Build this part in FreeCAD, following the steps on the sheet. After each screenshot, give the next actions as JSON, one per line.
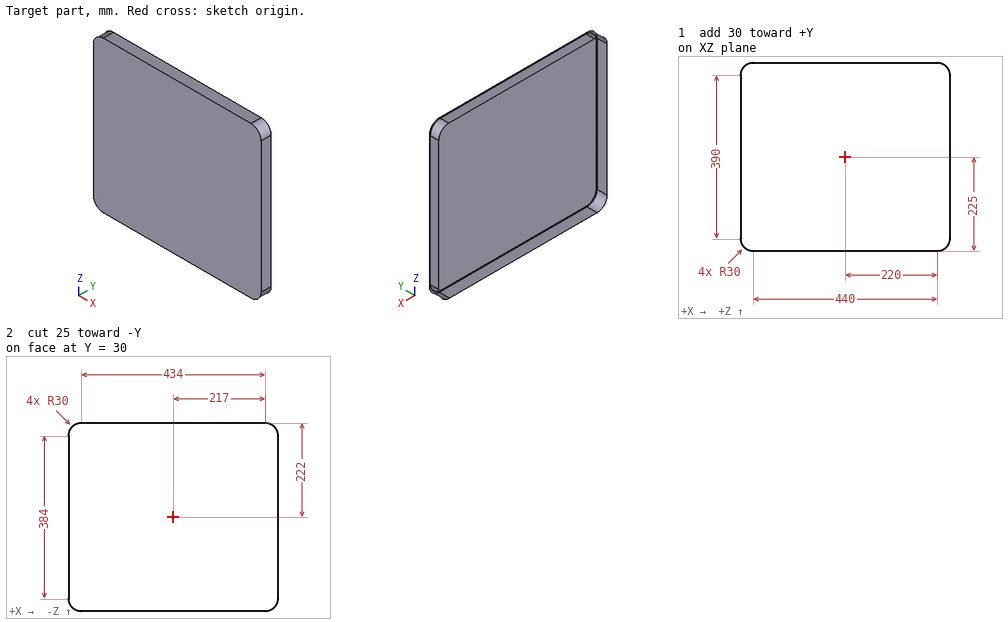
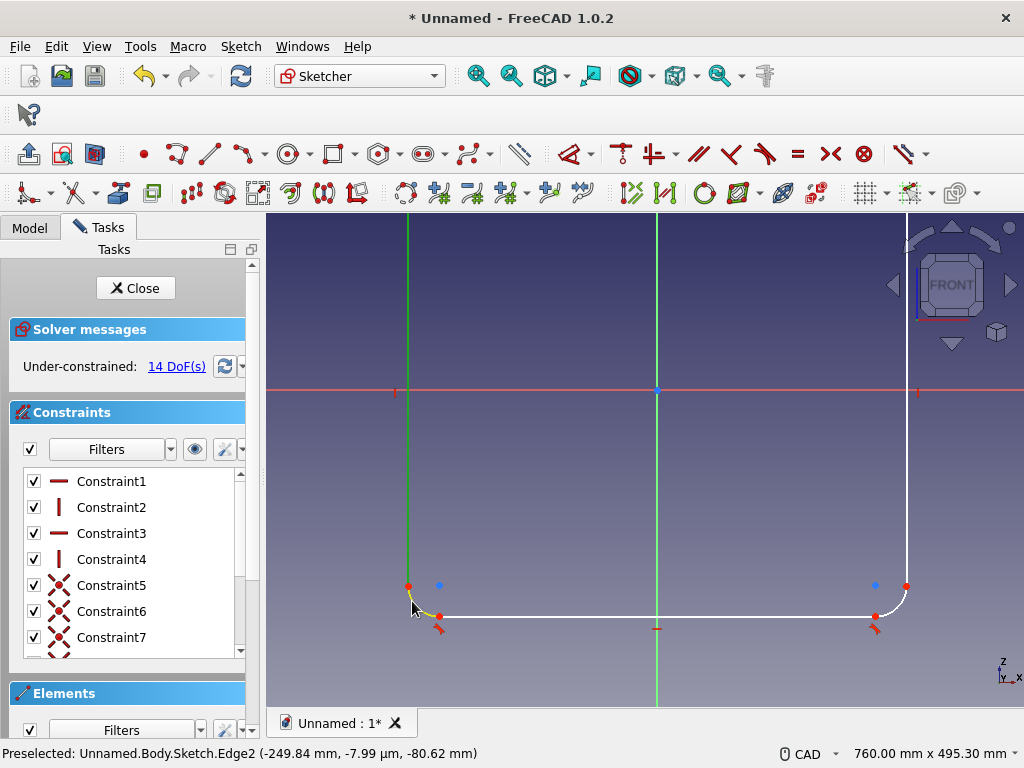
{"action": "left_click", "coordinate": [412, 600]}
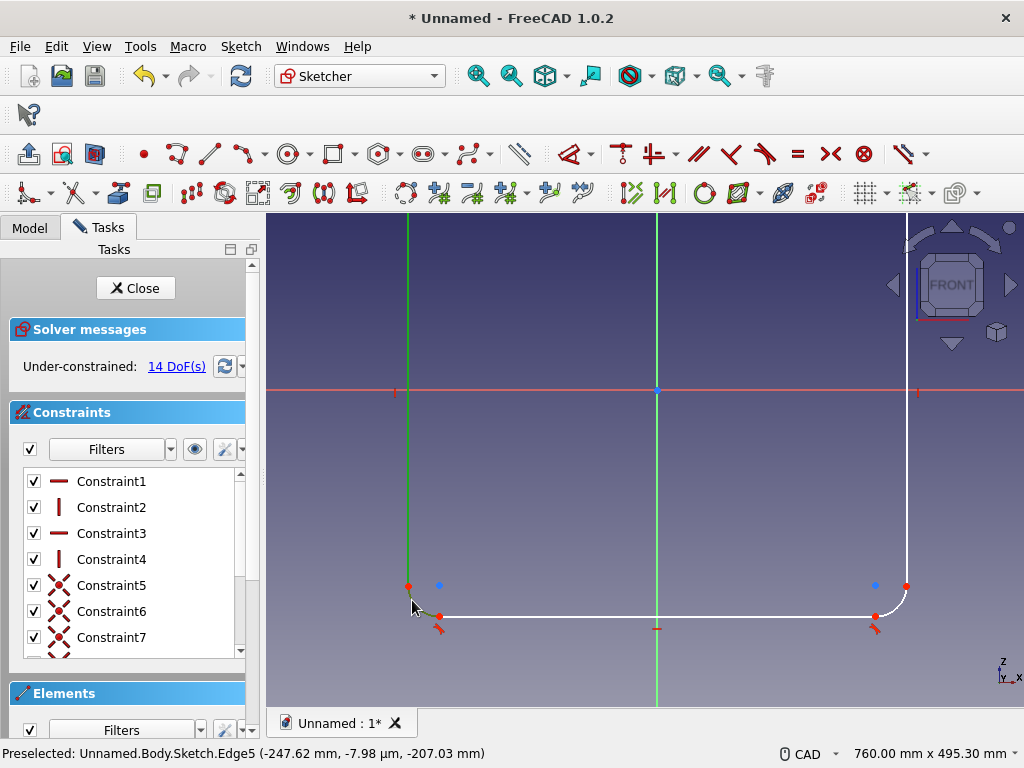
{"action": "left_click", "coordinate": [765, 154]}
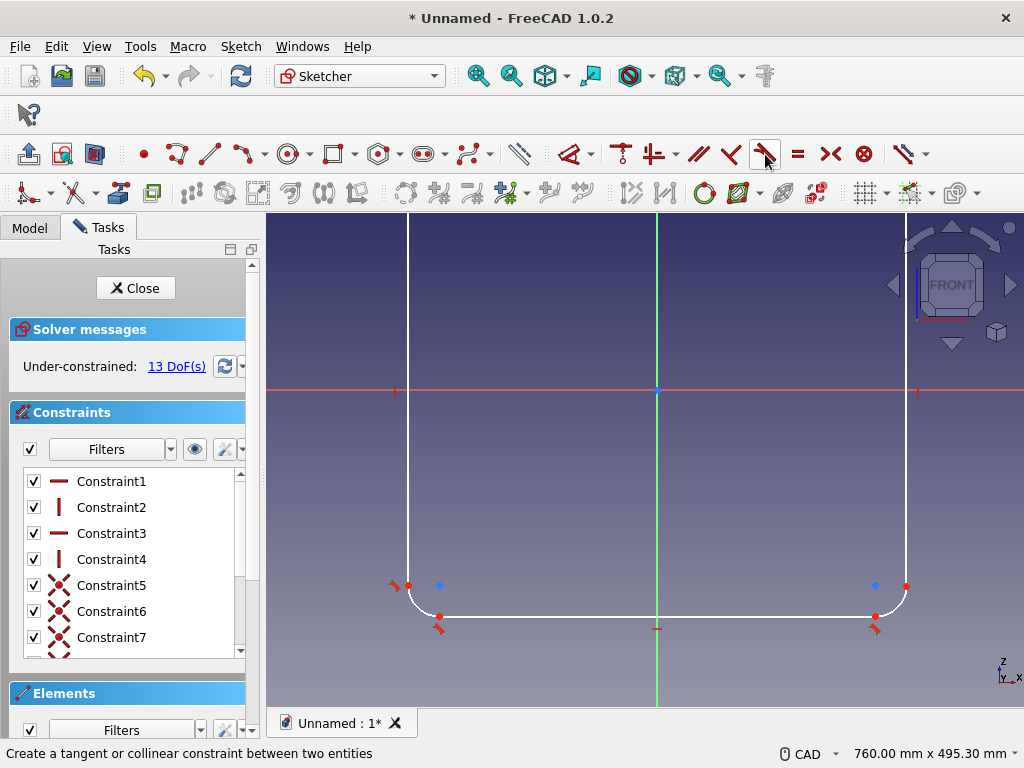
{"action": "left_click", "coordinate": [408, 469]}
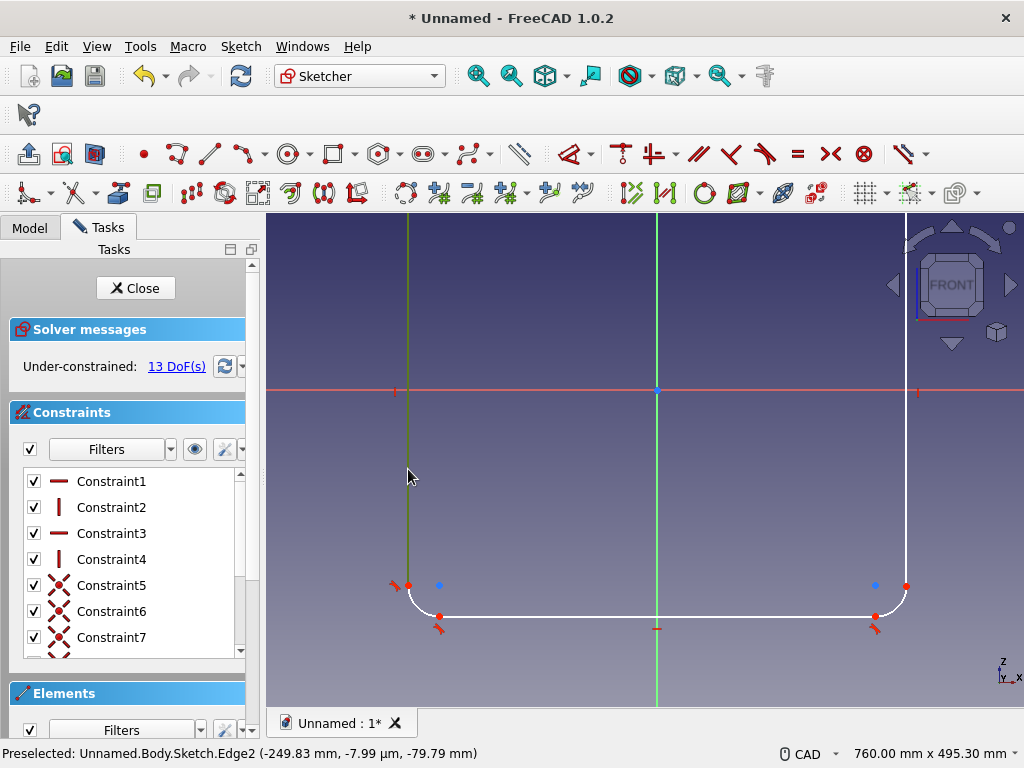
{"action": "scroll", "coordinate": [412, 601], "scroll_direction": "down", "scroll_amount": 2}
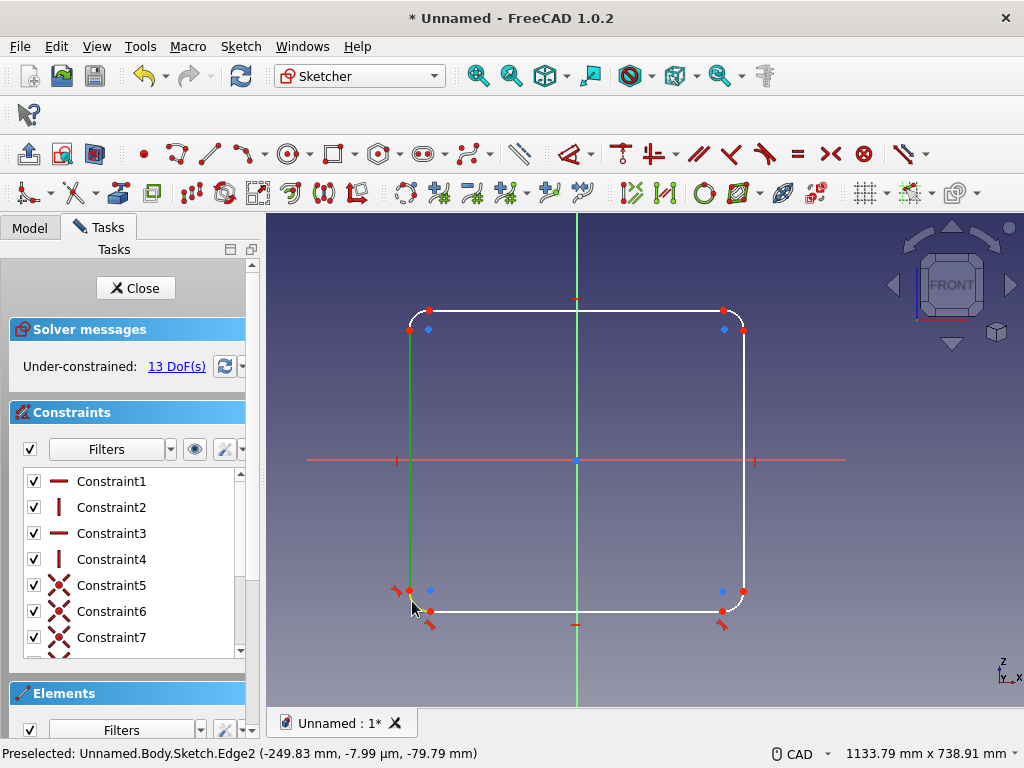
{"action": "scroll", "coordinate": [420, 312], "scroll_direction": "up", "scroll_amount": 2}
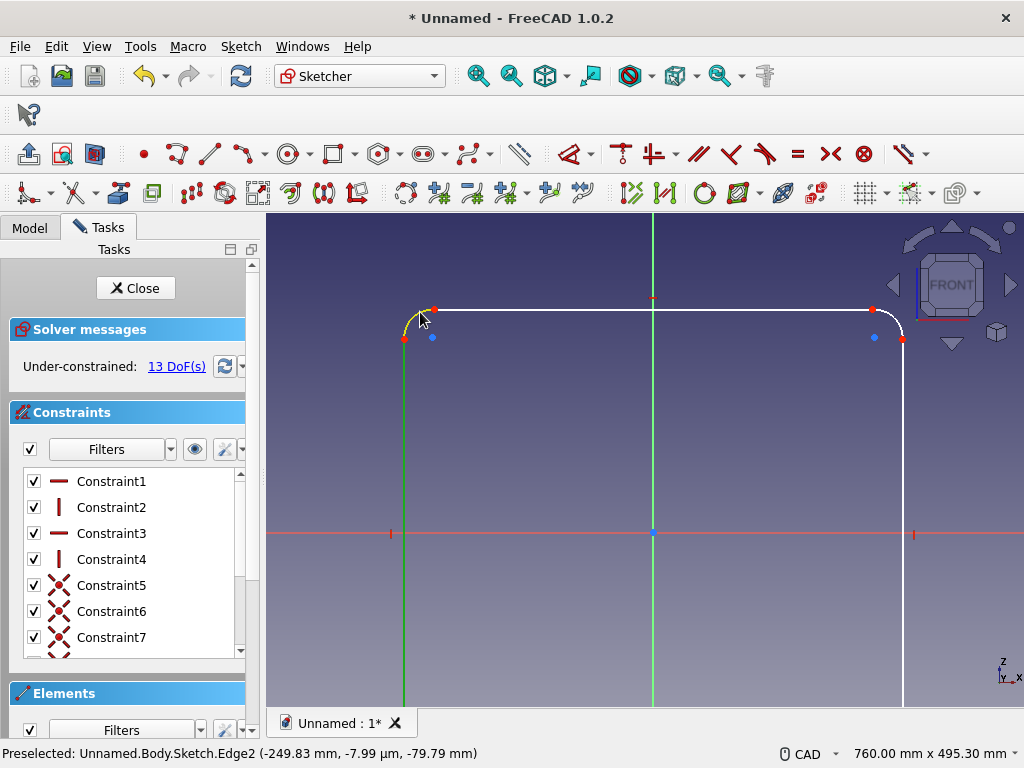
{"action": "left_click", "coordinate": [420, 313]}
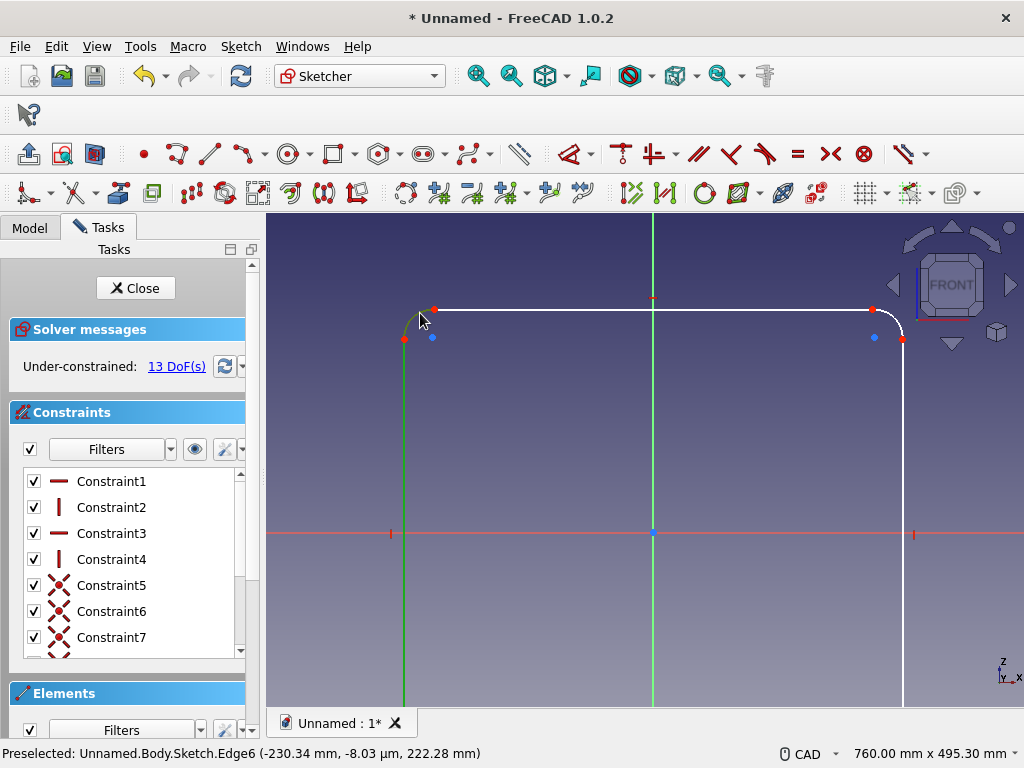
{"action": "left_click", "coordinate": [765, 154]}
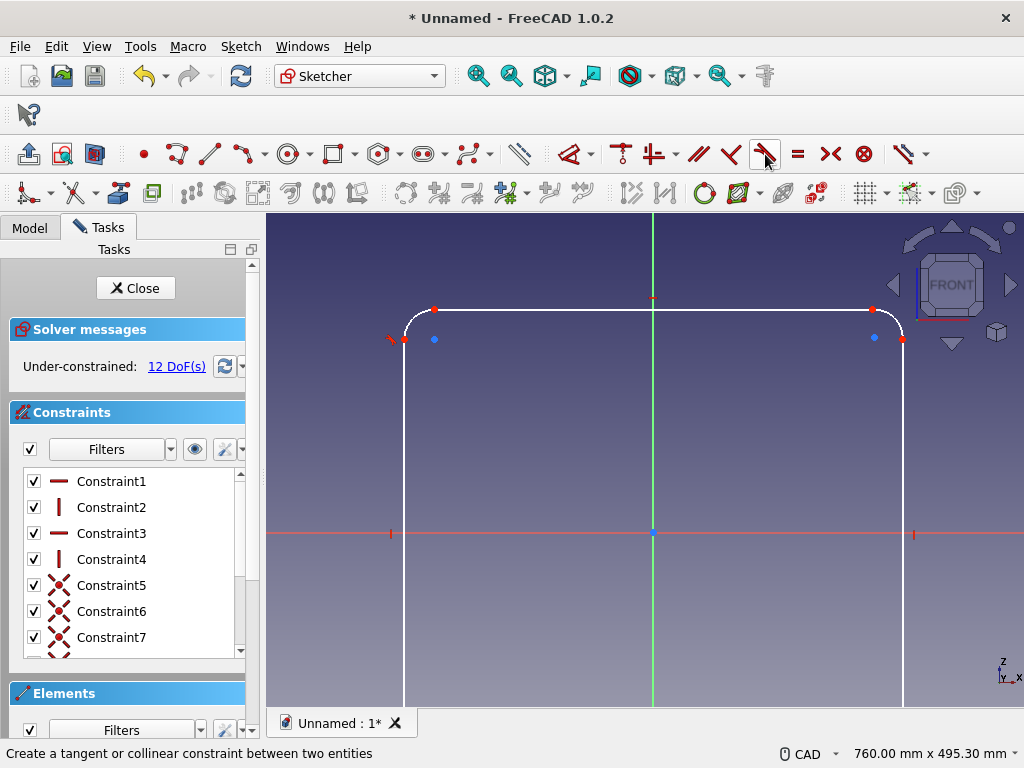
{"action": "left_click", "coordinate": [566, 310]}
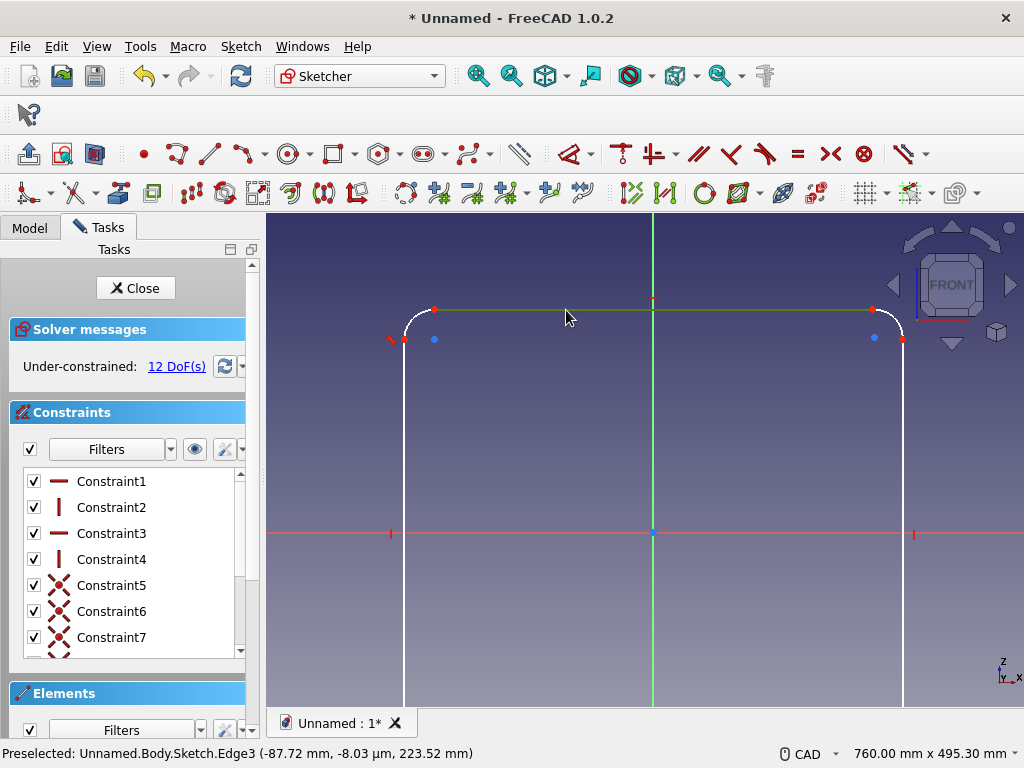
{"action": "left_click", "coordinate": [421, 313]}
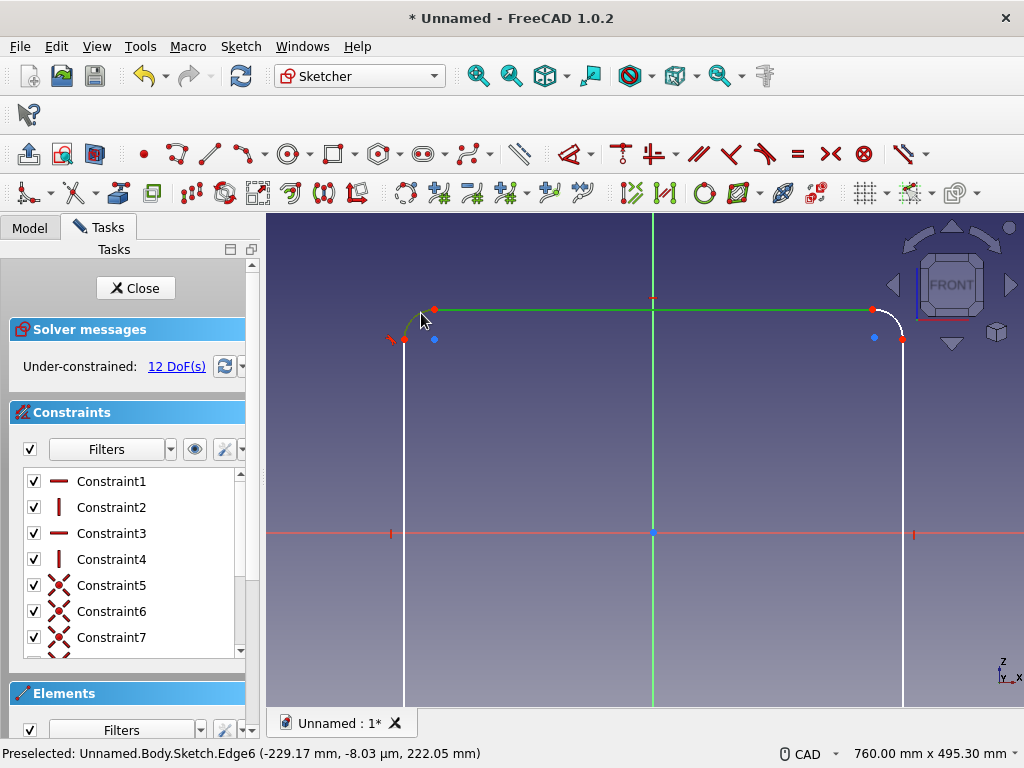
{"action": "left_click", "coordinate": [765, 154]}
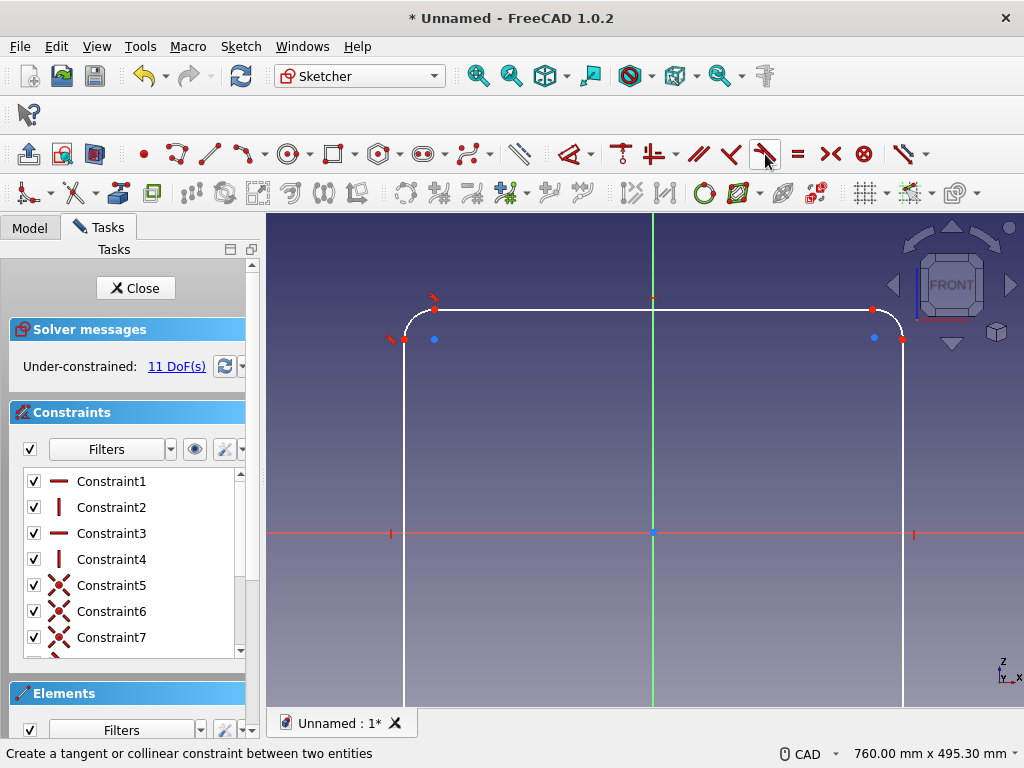
{"action": "left_click", "coordinate": [566, 310]}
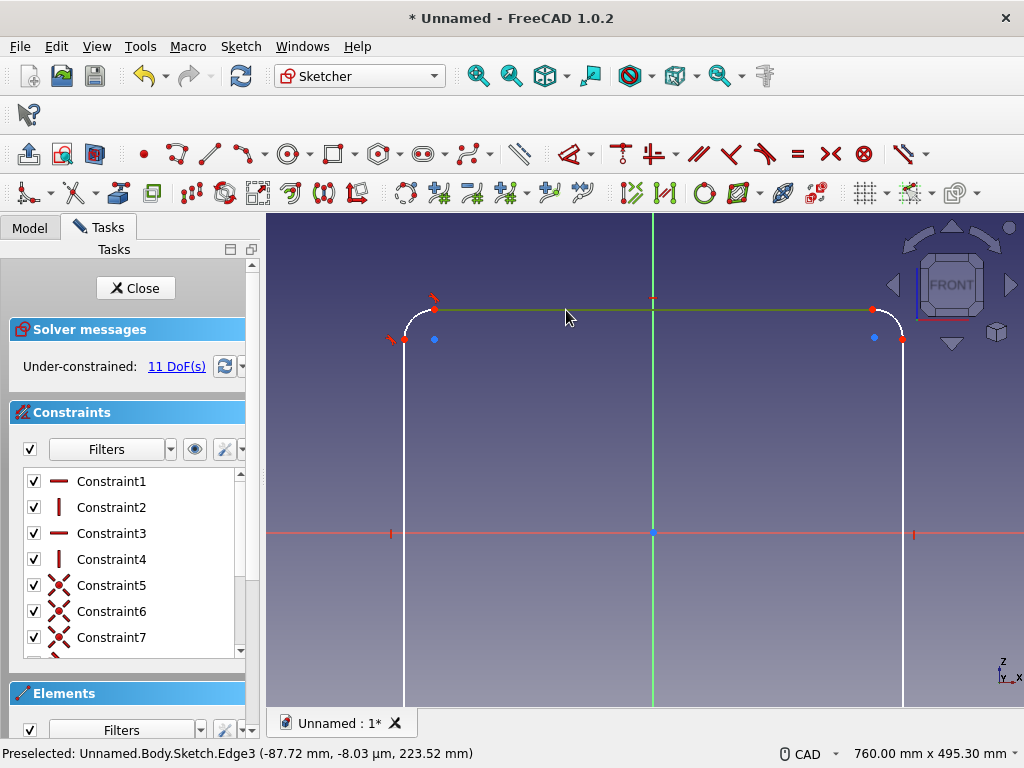
{"action": "scroll", "coordinate": [420, 312], "scroll_direction": "down", "scroll_amount": 2}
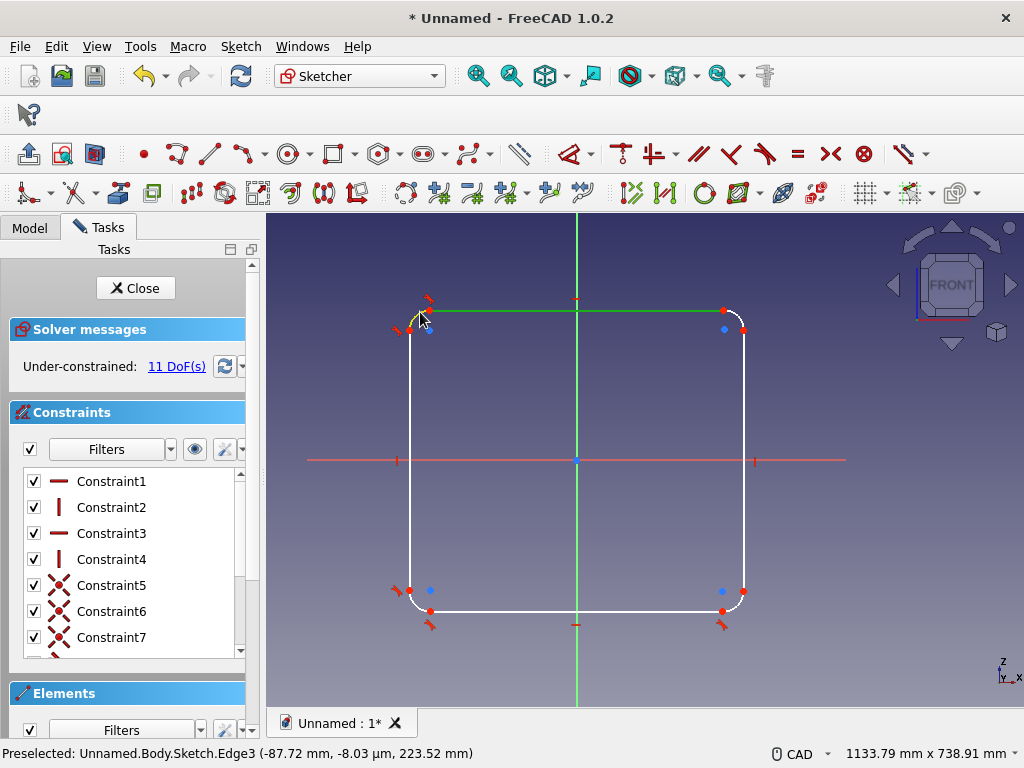
{"action": "scroll", "coordinate": [742, 321], "scroll_direction": "up", "scroll_amount": 2}